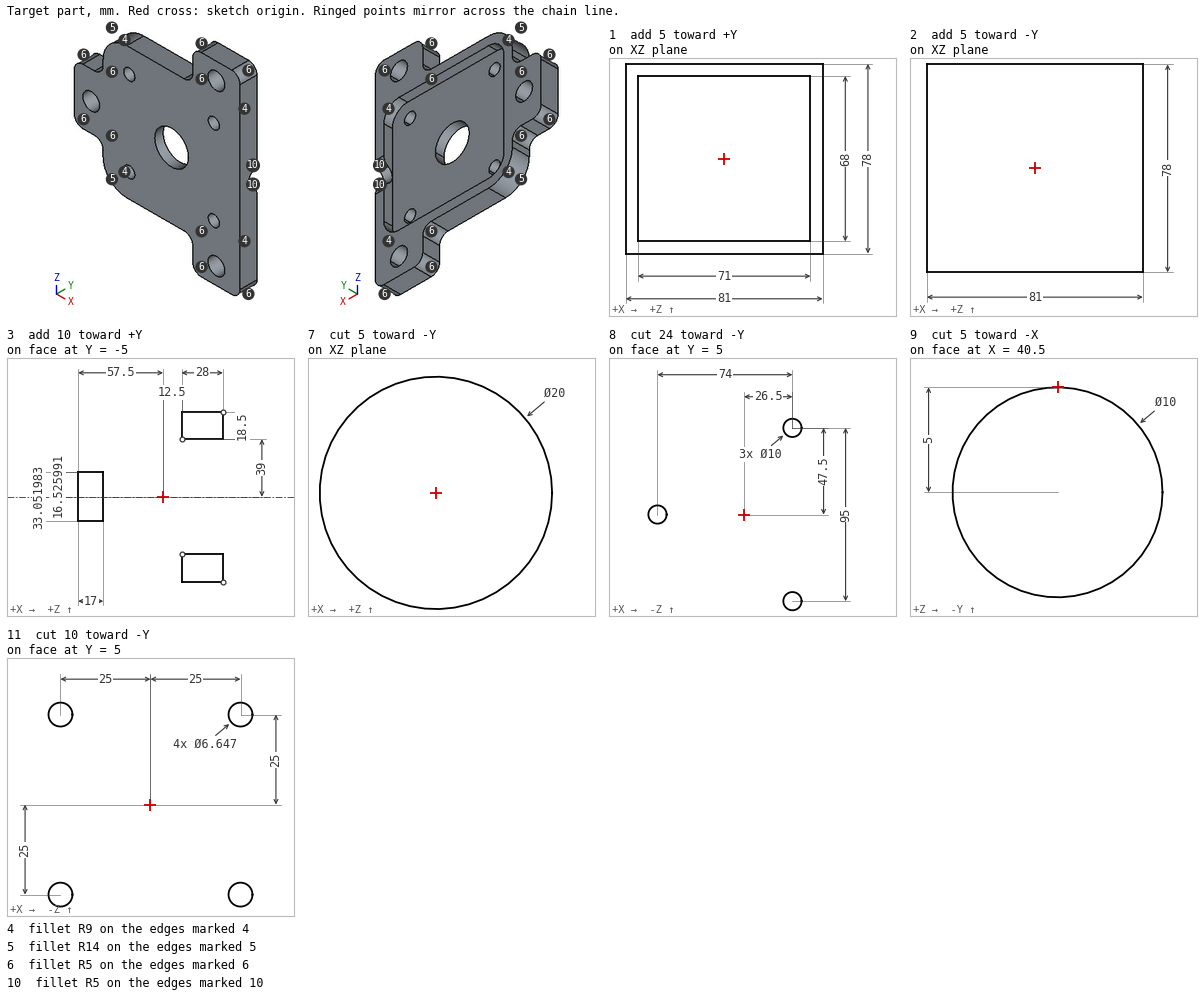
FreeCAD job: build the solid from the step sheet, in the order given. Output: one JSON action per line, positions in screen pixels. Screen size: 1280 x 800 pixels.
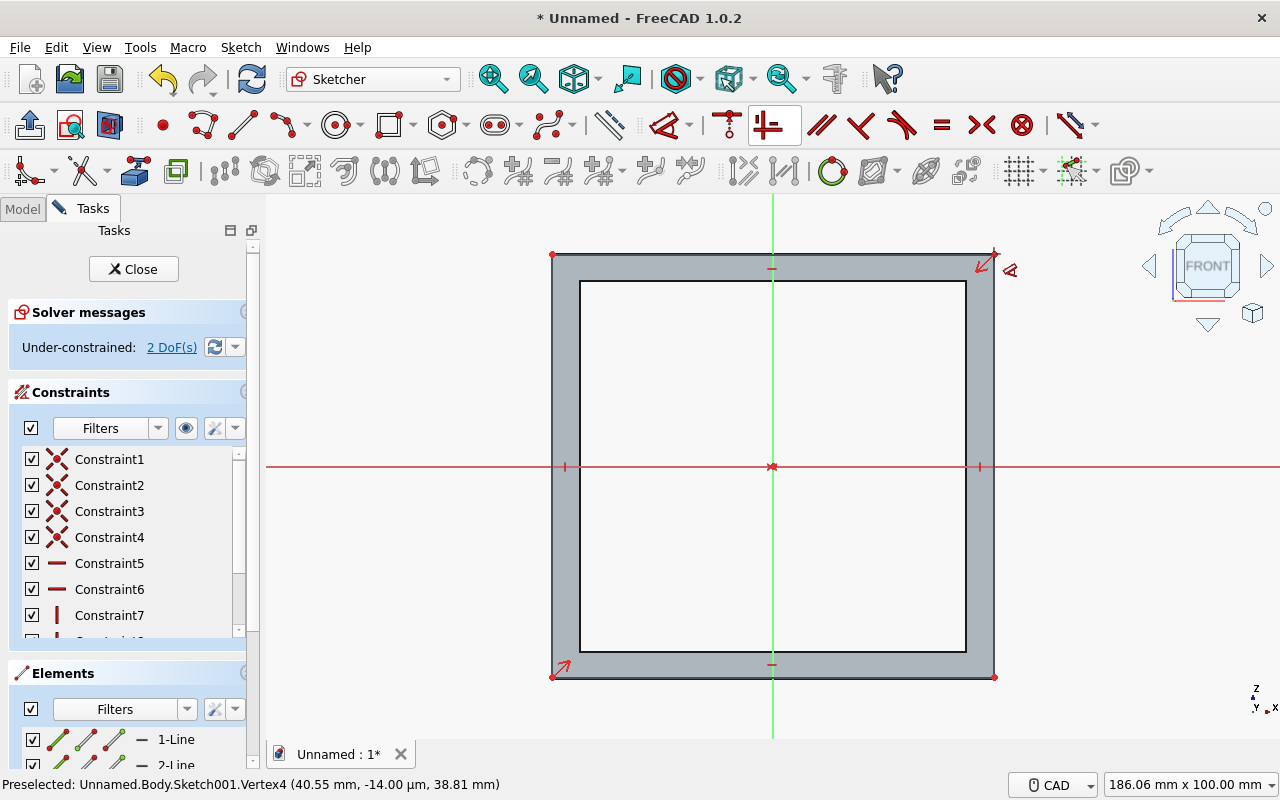
{"action": "left_click", "coordinate": [685, 678]}
{"action": "left_click", "coordinate": [671, 644]}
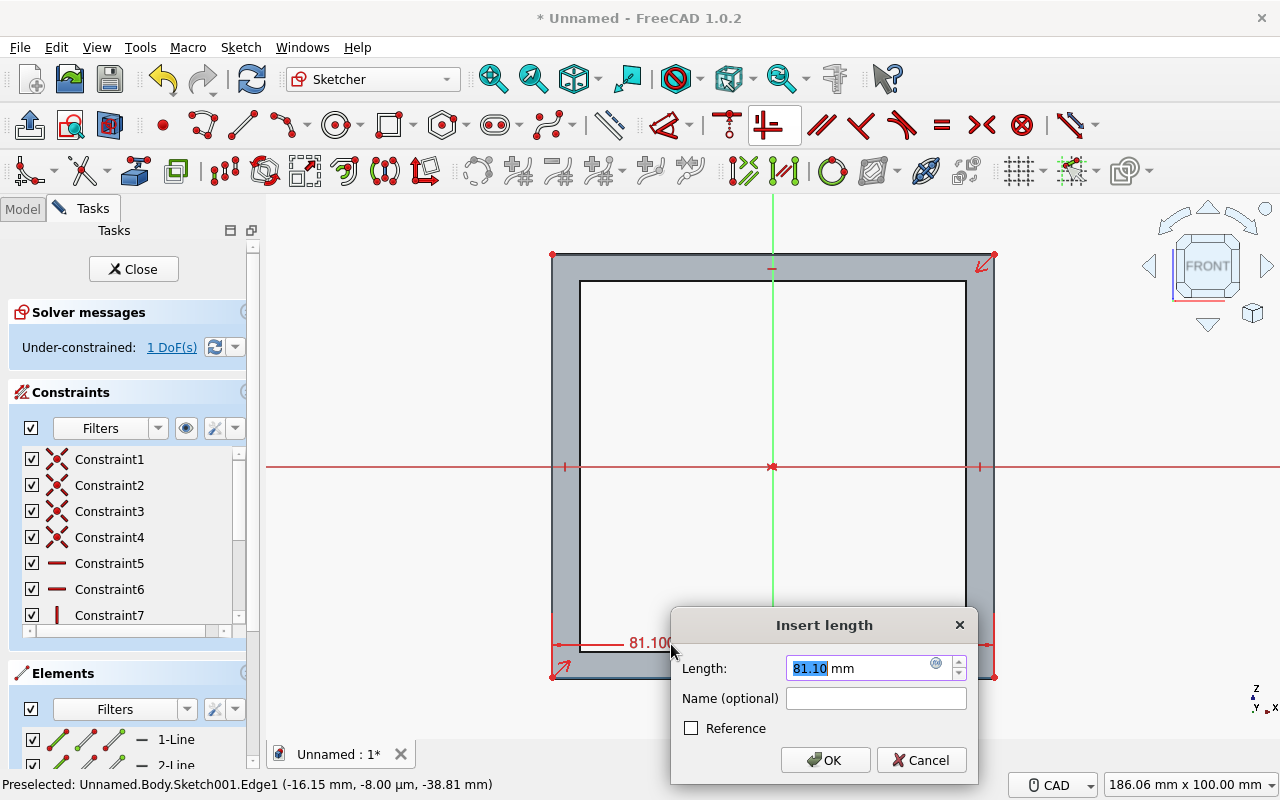
{"action": "type", "text": "81"}
{"action": "key", "text": "Return"}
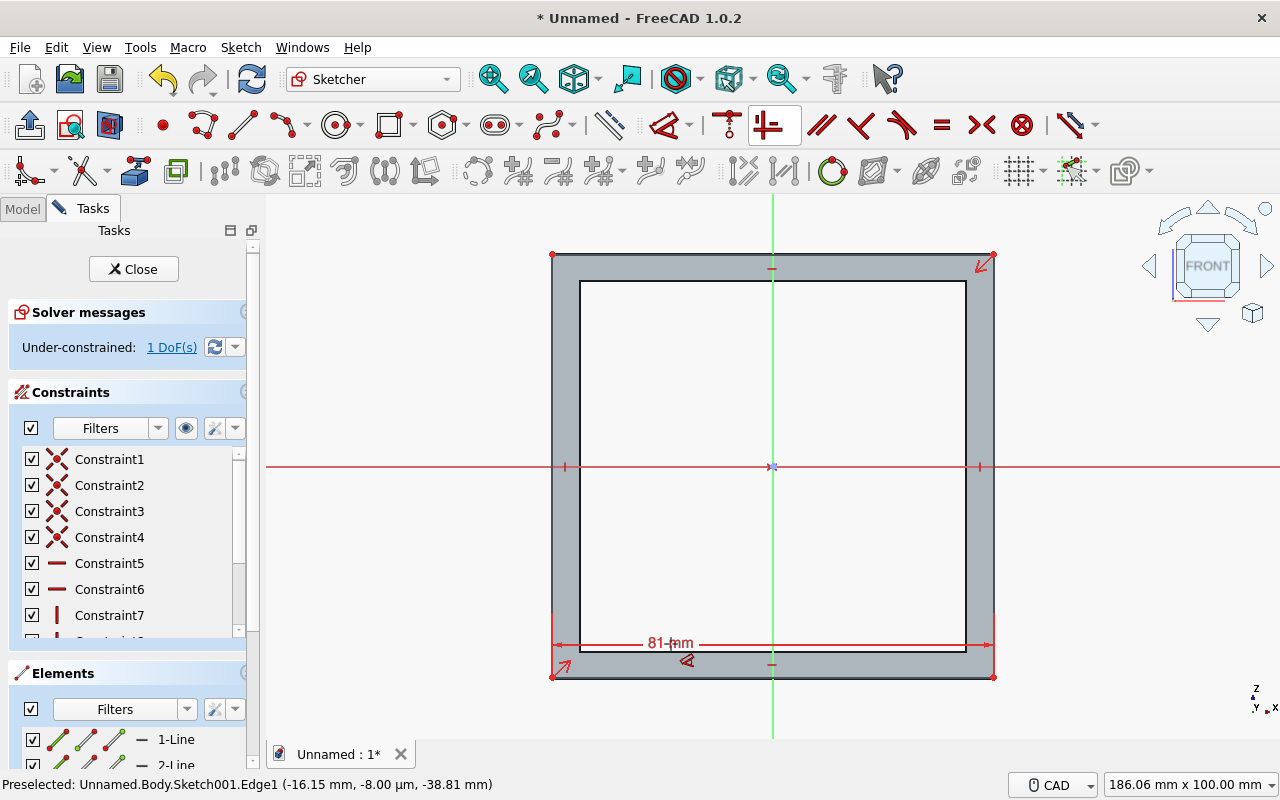
{"action": "left_click", "coordinate": [994, 551]}
{"action": "left_click", "coordinate": [1028, 369]}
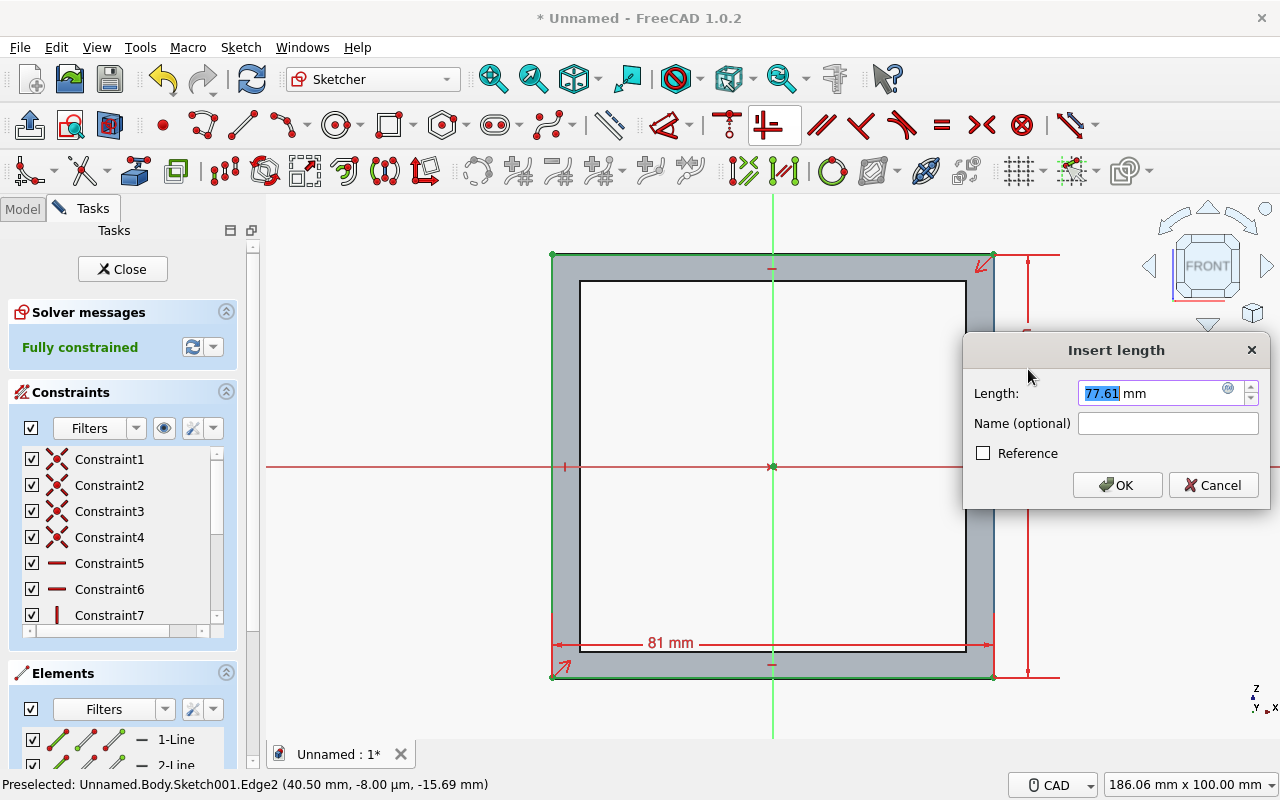
{"action": "type", "text": "78"}
{"action": "key", "text": "Return"}
{"action": "key", "text": "Escape"}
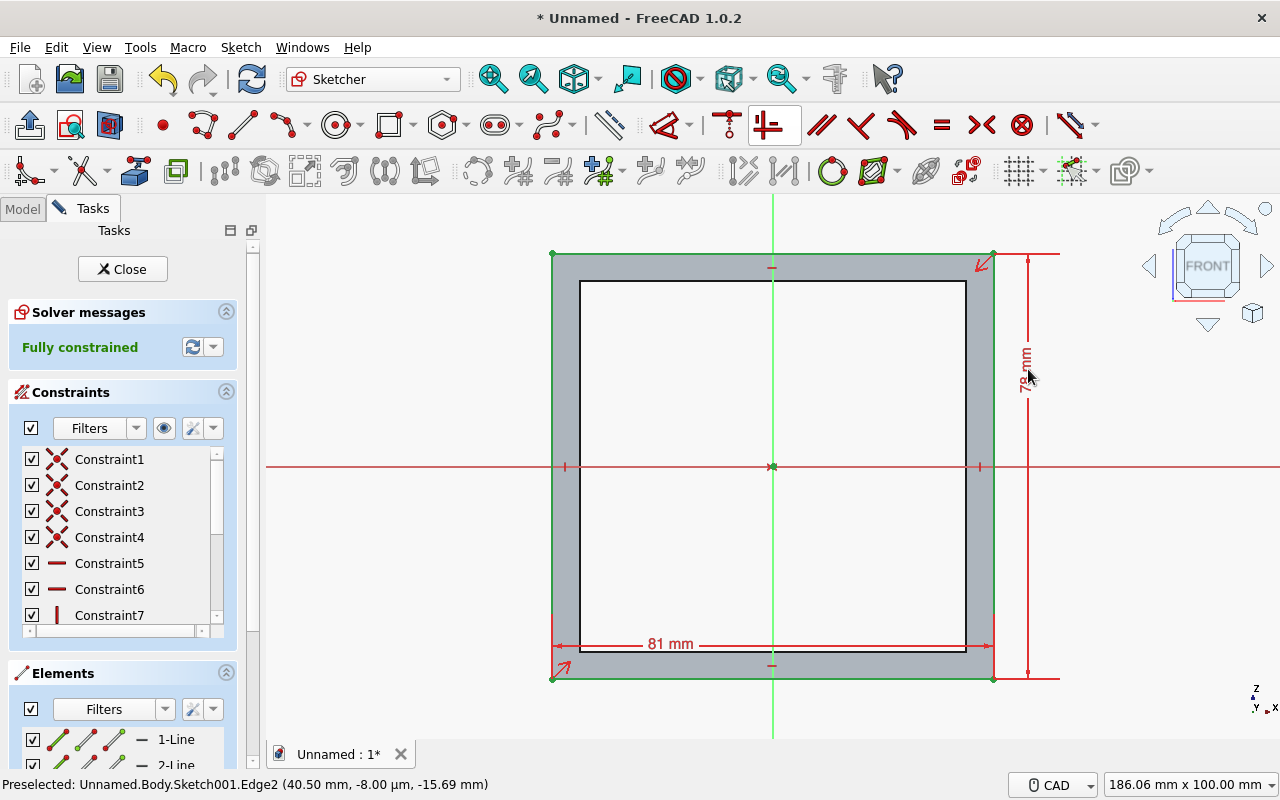
{"action": "left_click", "coordinate": [123, 269]}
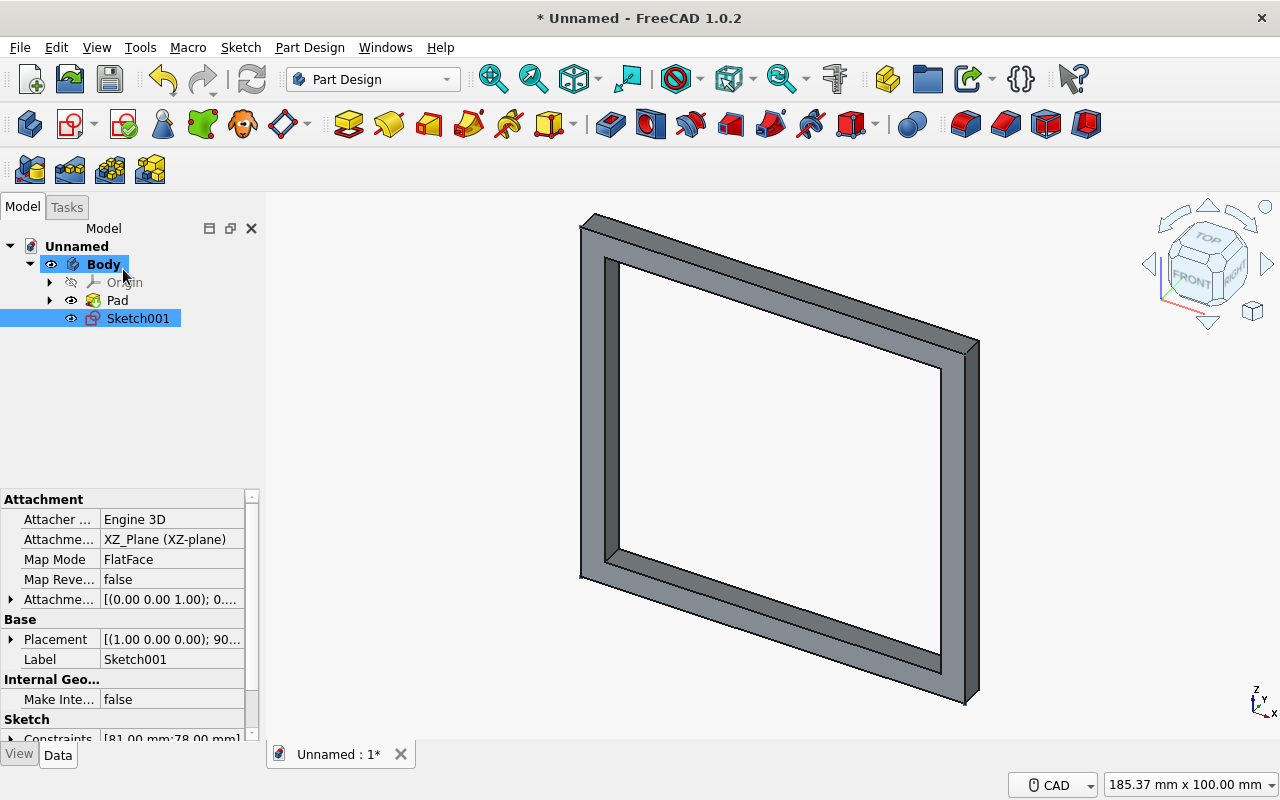
{"action": "left_click", "coordinate": [350, 124]}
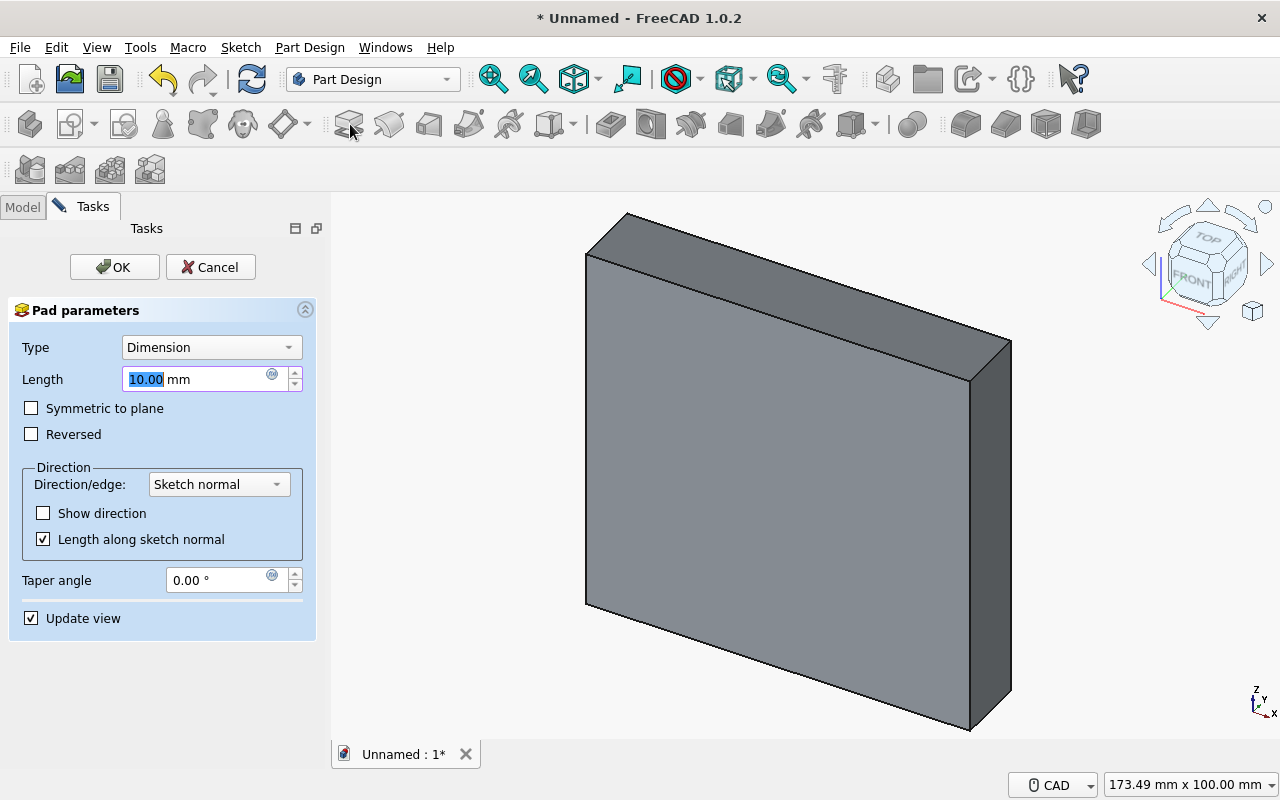
{"action": "type", "text": "5"}
{"action": "key", "text": "Tab"}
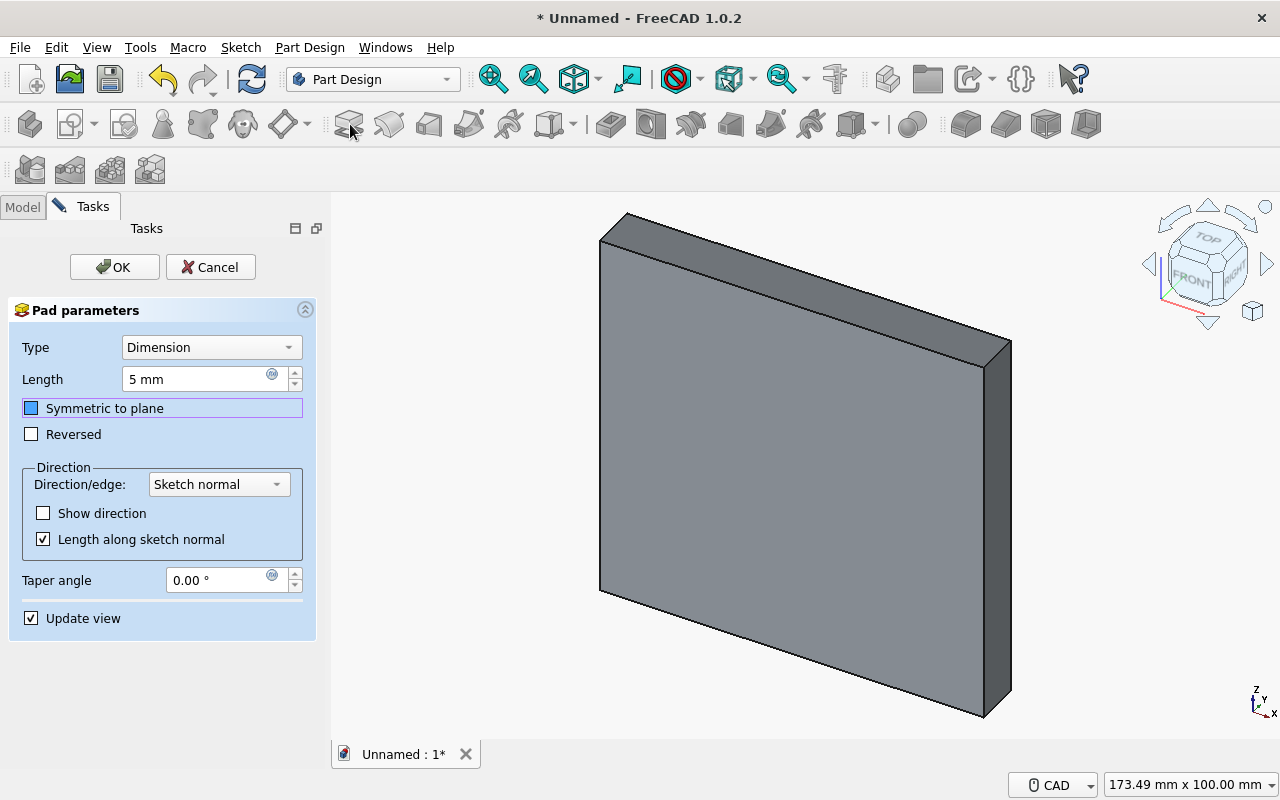
{"action": "left_click", "coordinate": [115, 267]}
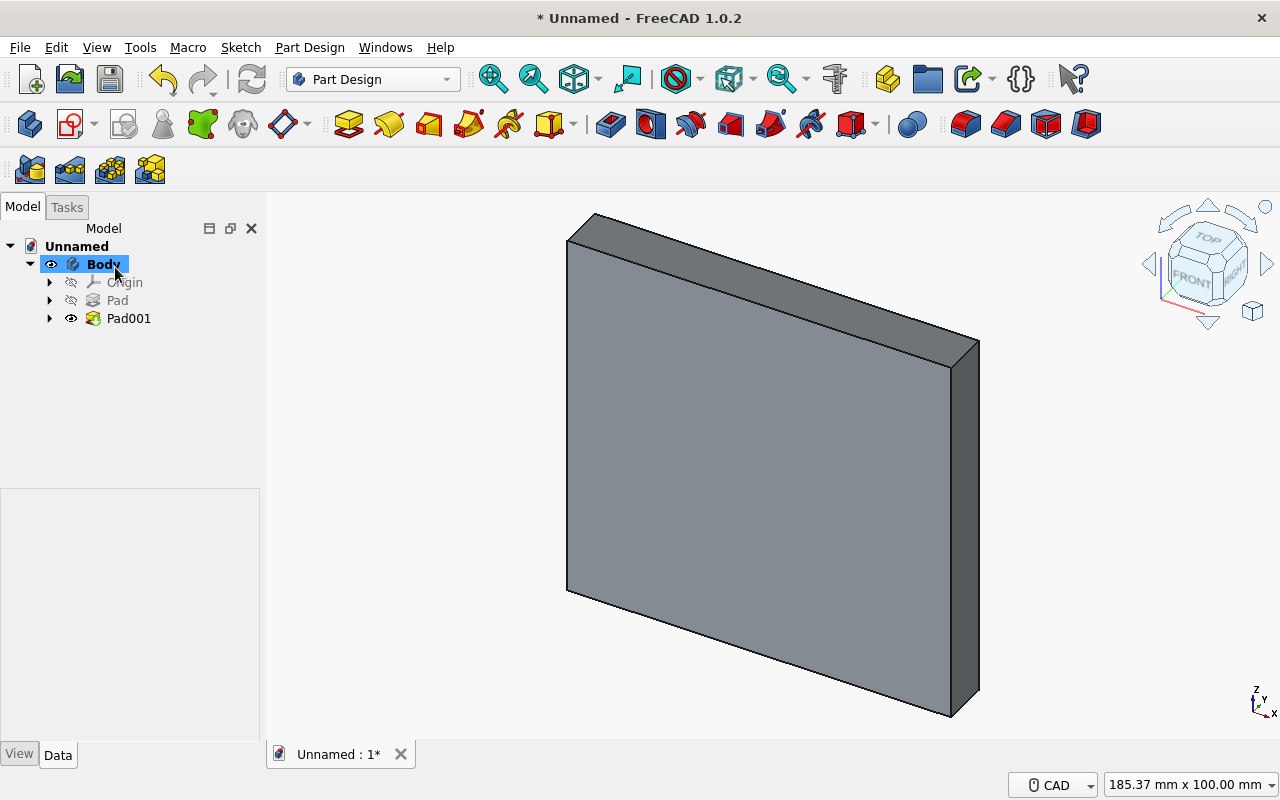
{"action": "left_click", "coordinate": [759, 478]}